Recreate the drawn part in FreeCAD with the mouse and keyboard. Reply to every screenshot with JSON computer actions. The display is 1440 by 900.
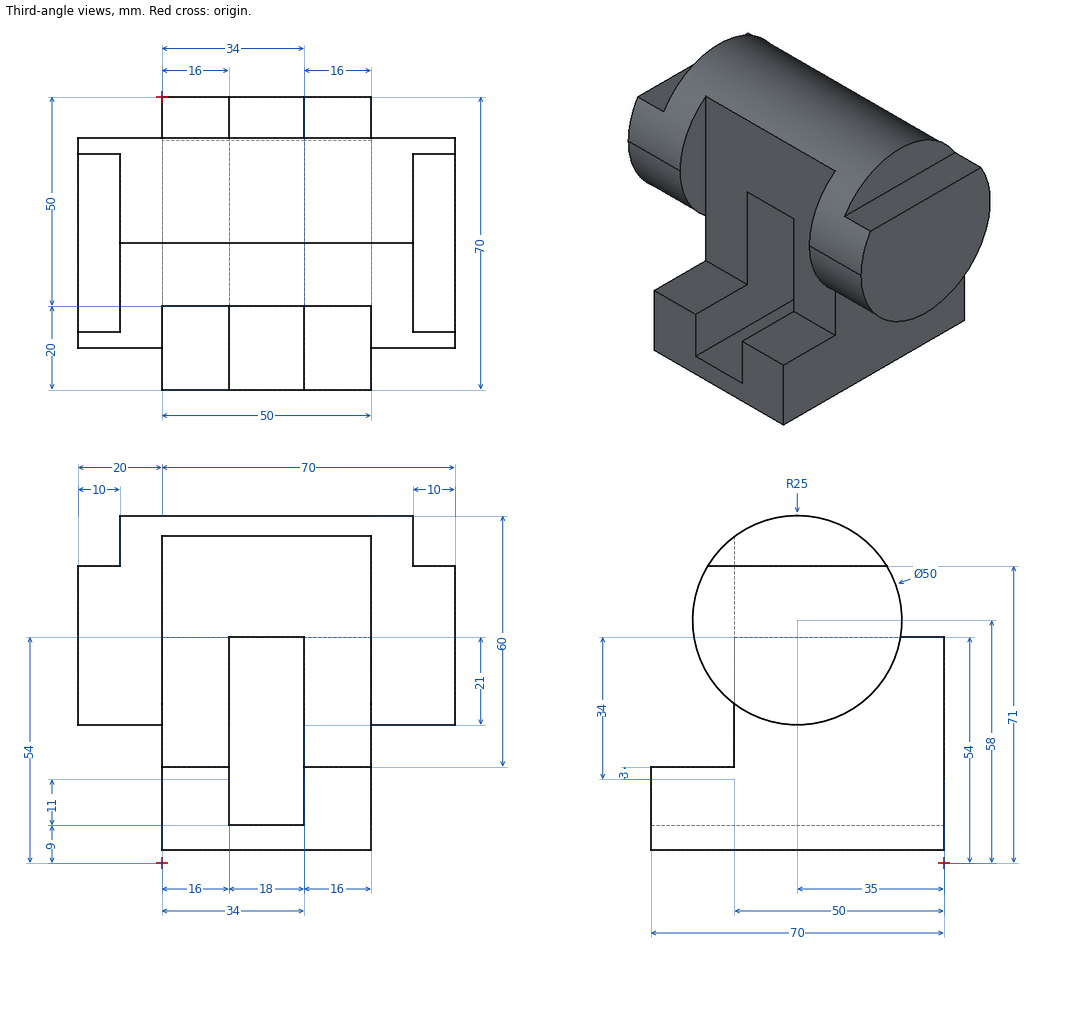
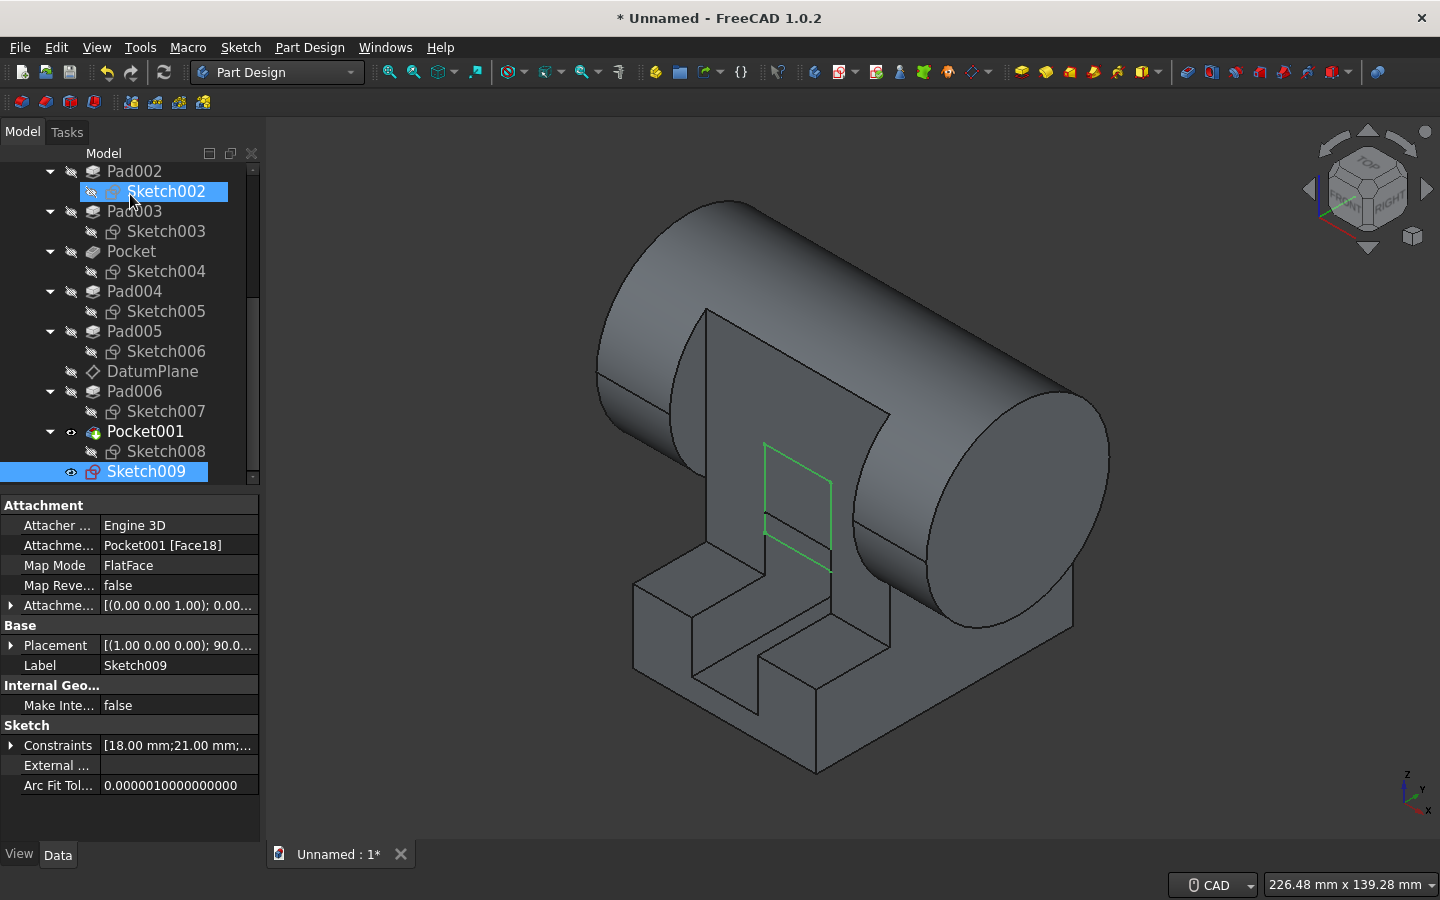
{"action": "left_click", "coordinate": [1188, 72]}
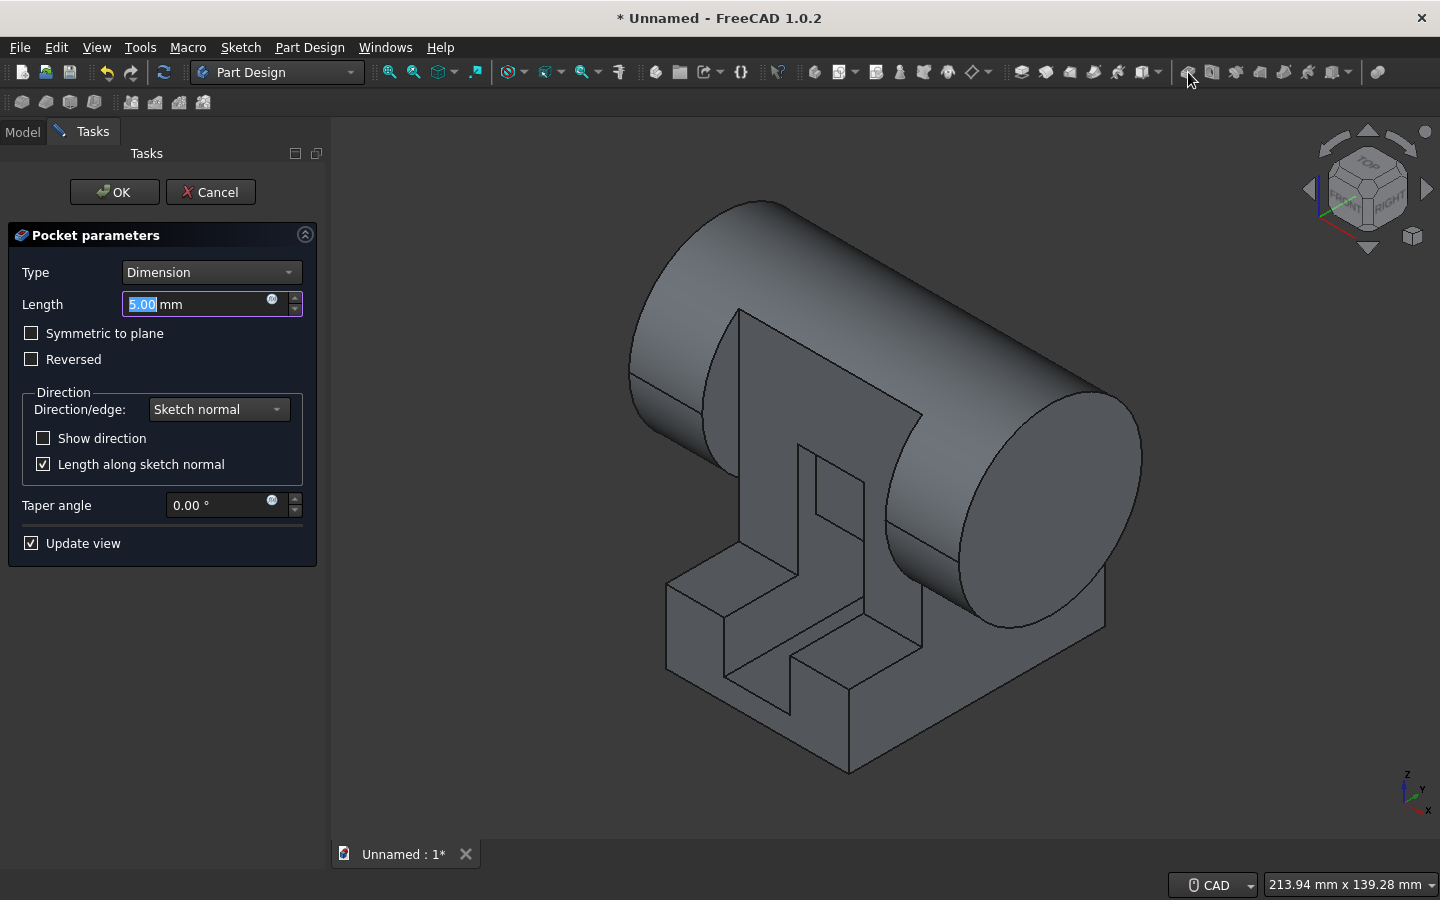
{"action": "type", "text": "50"}
{"action": "key", "text": "Tab"}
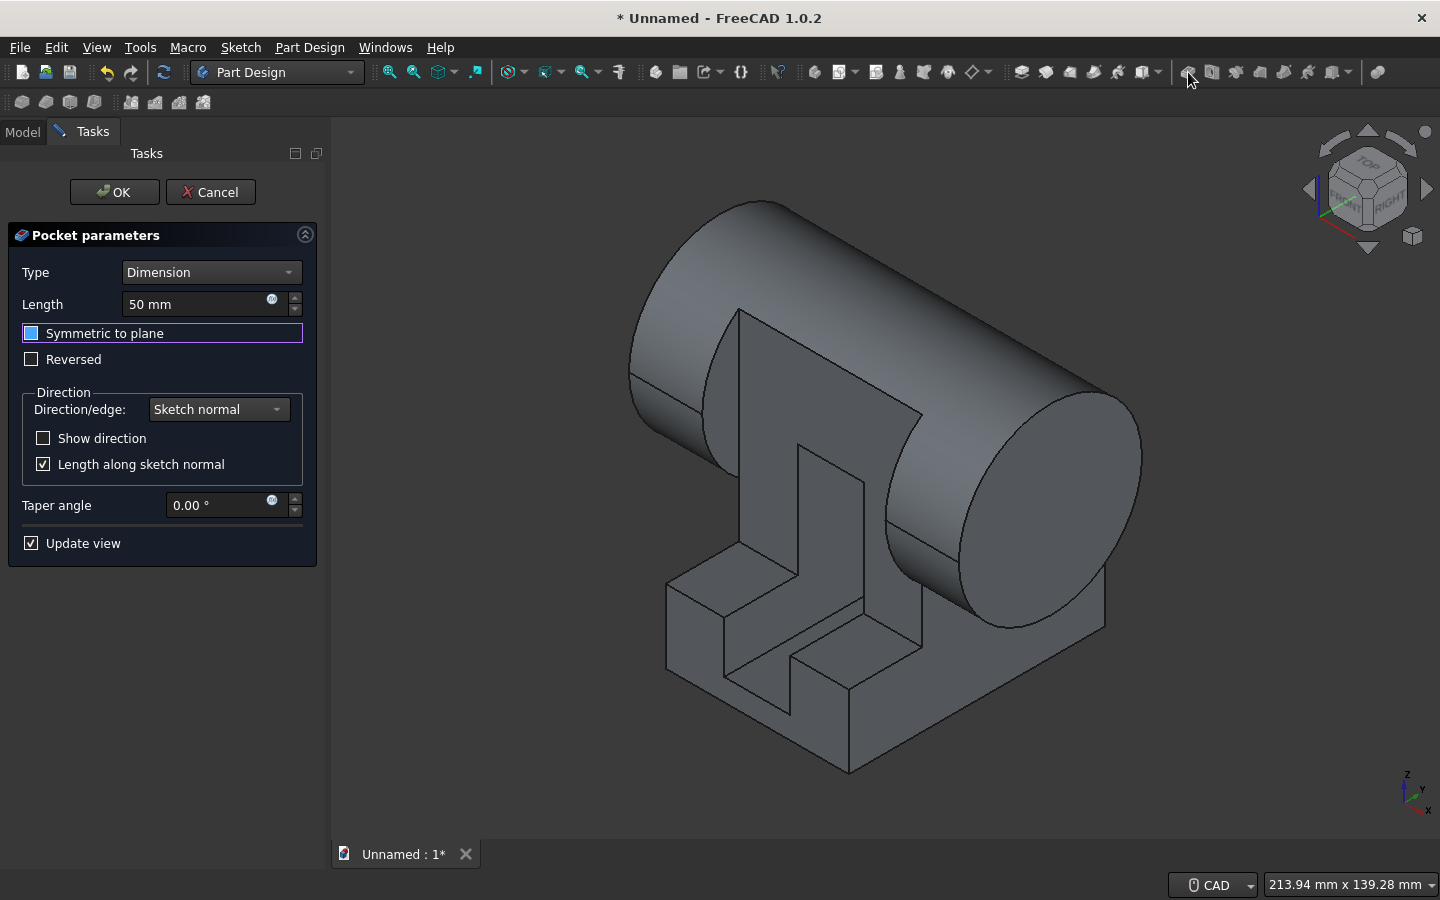
{"action": "left_click", "coordinate": [115, 192]}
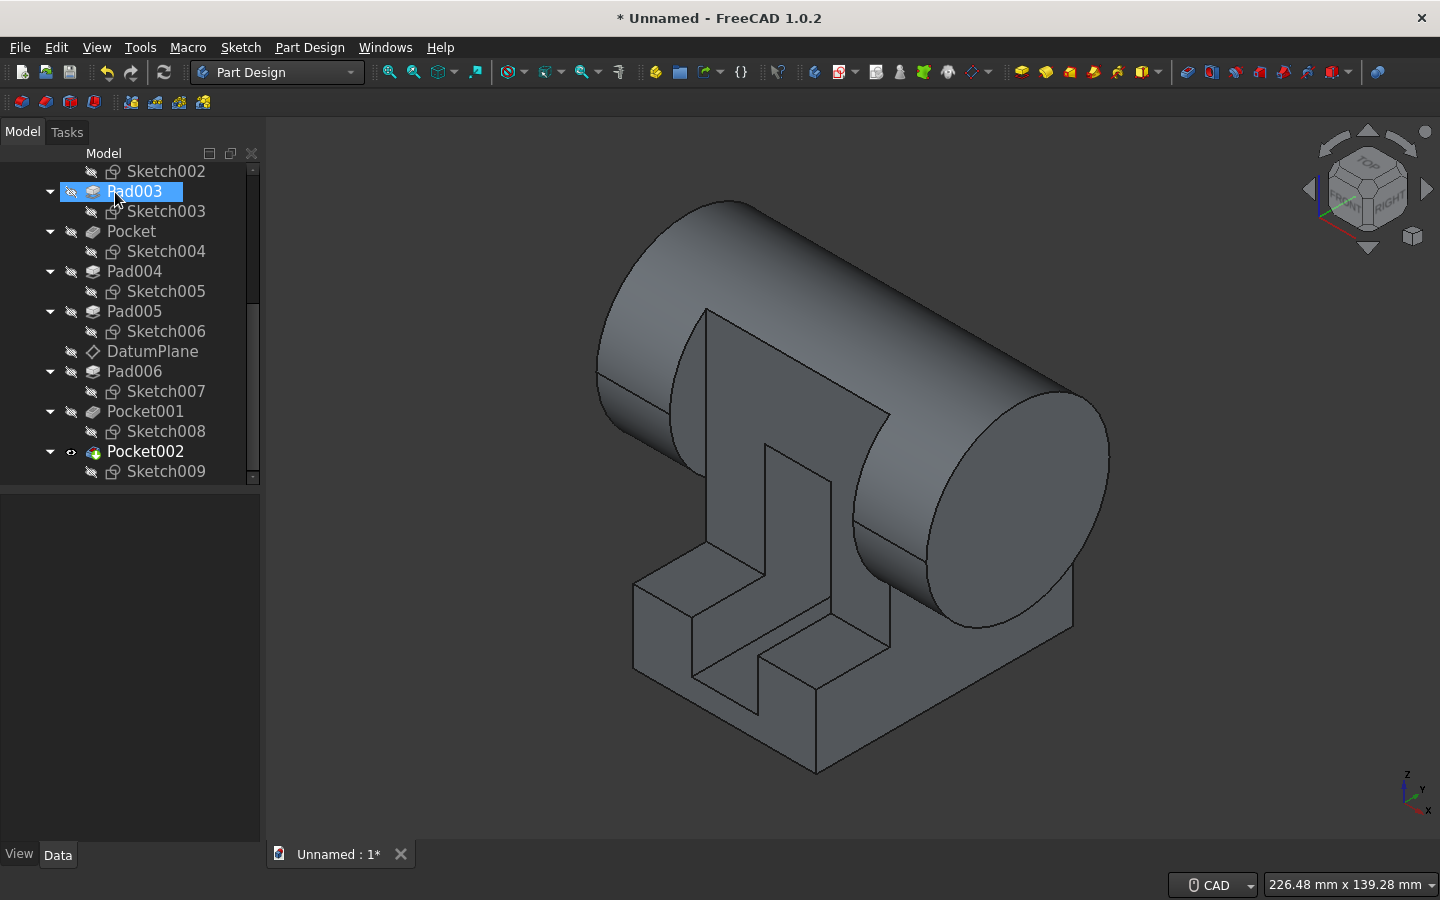
{"action": "key", "text": "6"}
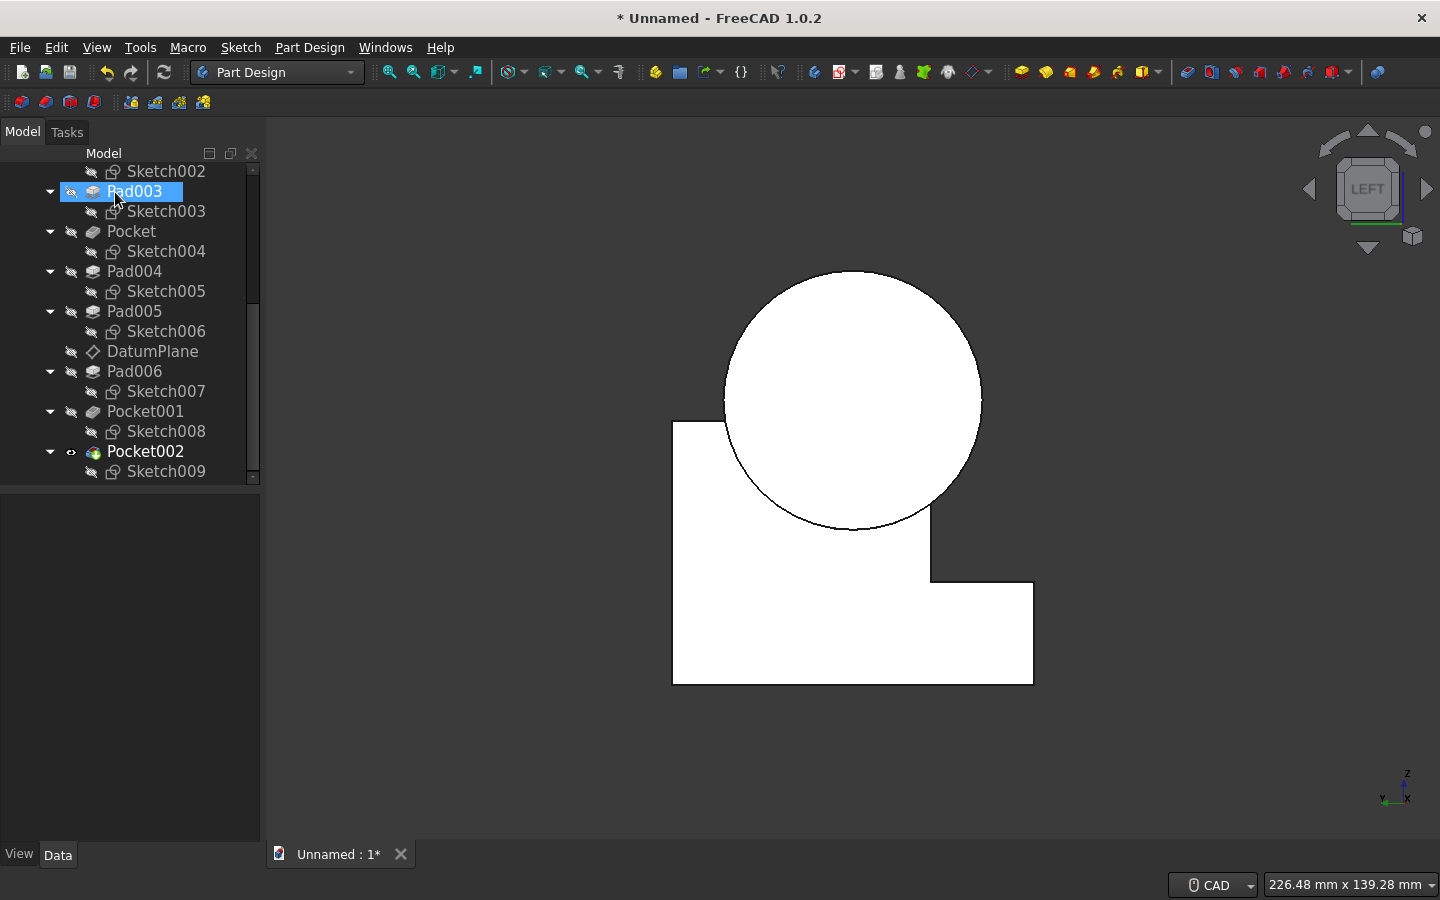
{"action": "left_click", "coordinate": [853, 399]}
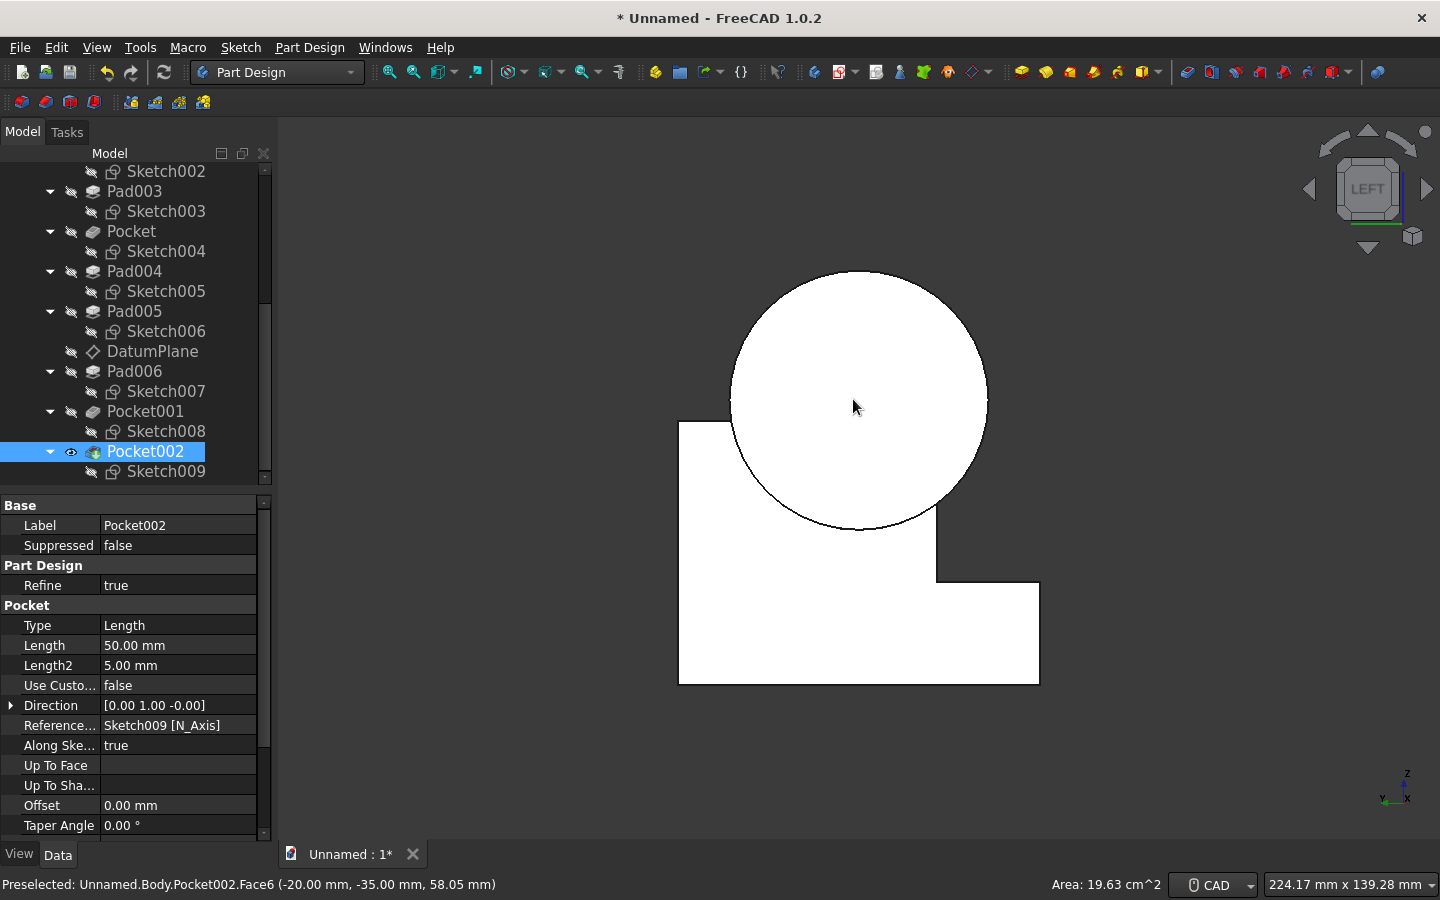
{"action": "left_click", "coordinate": [840, 72]}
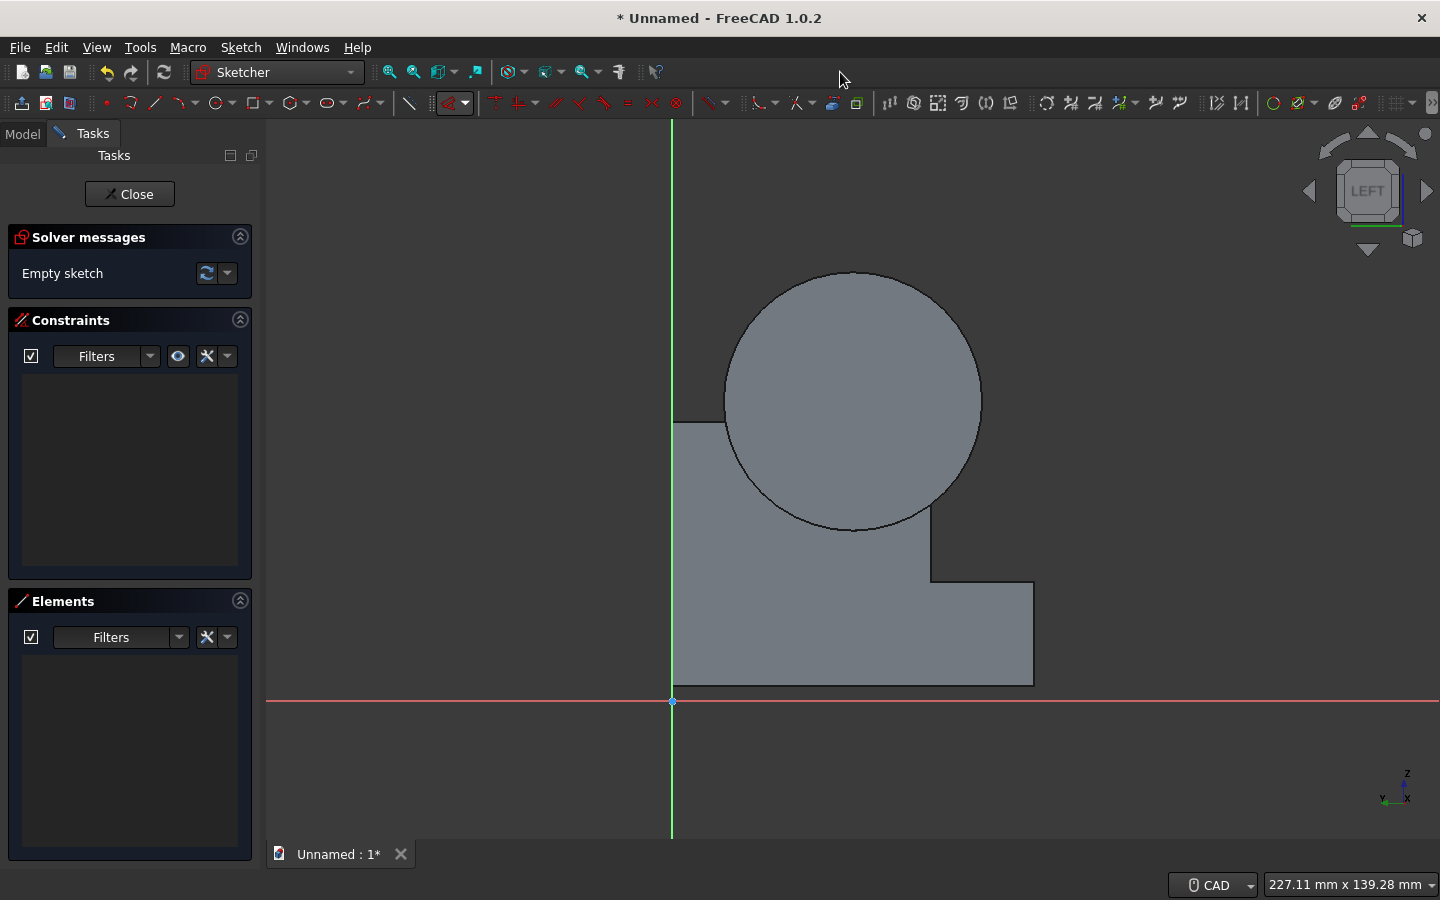
{"action": "key", "text": "g l"}